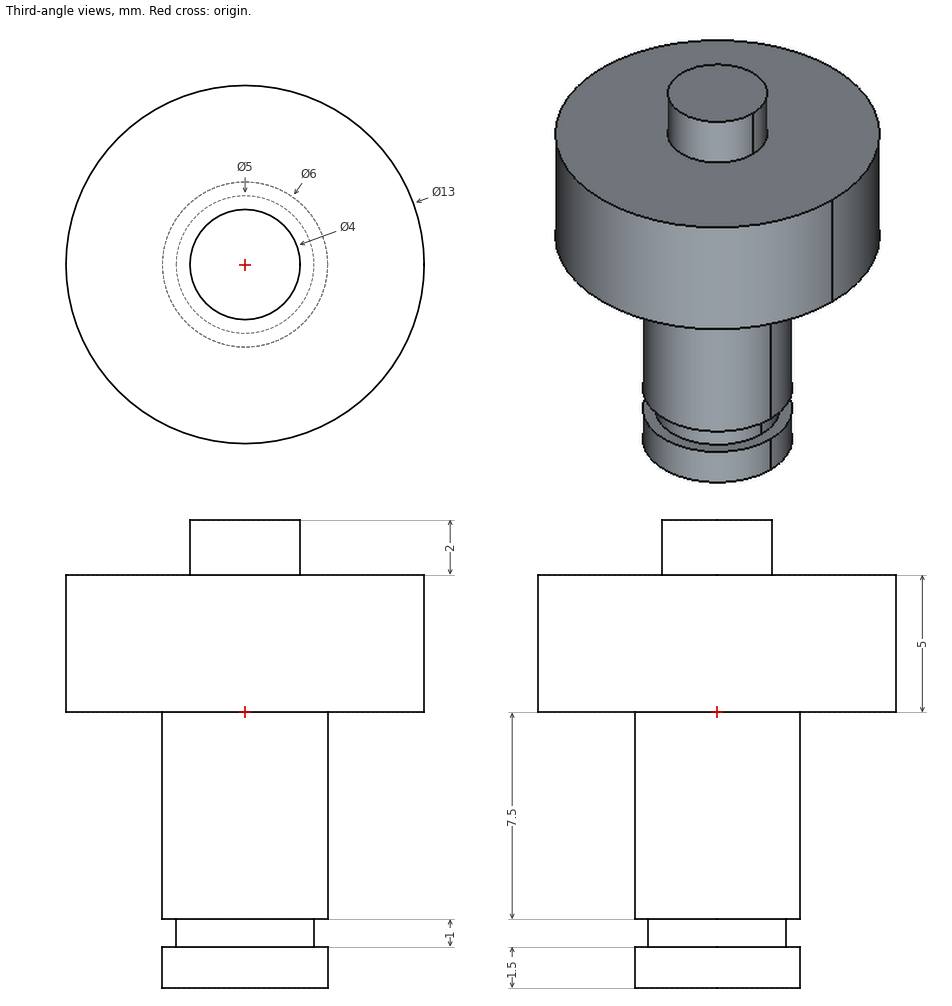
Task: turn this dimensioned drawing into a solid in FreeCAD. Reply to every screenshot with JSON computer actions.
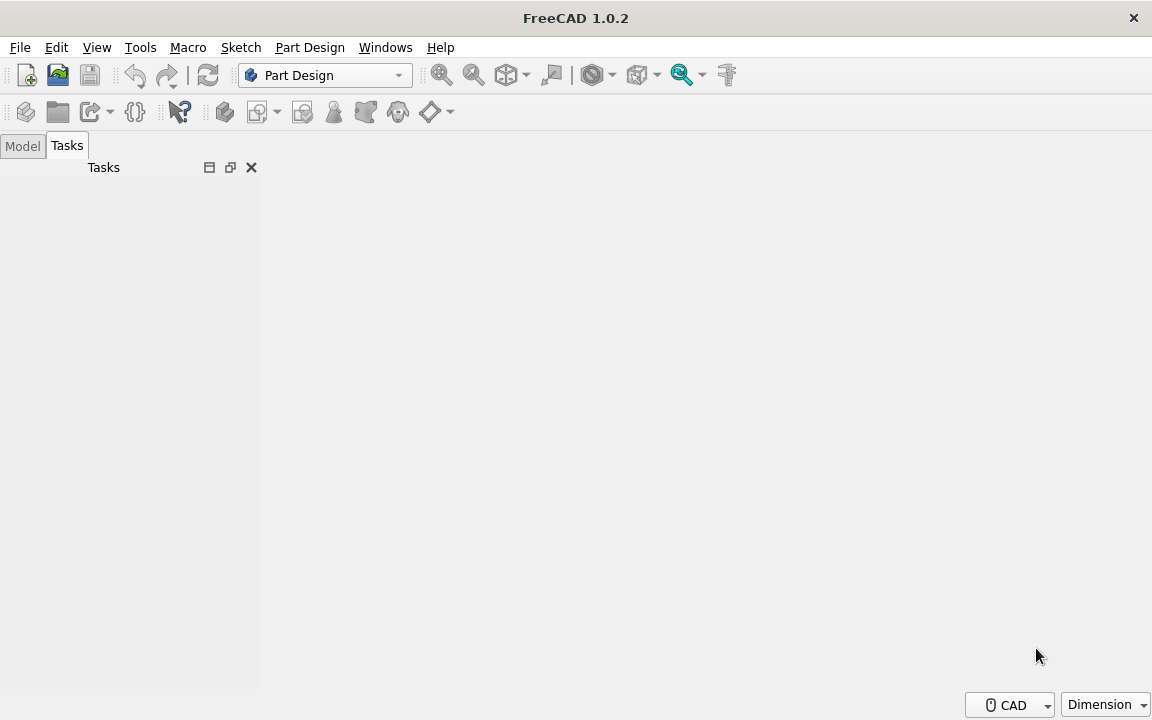
{"action": "key", "text": "ctrl+n"}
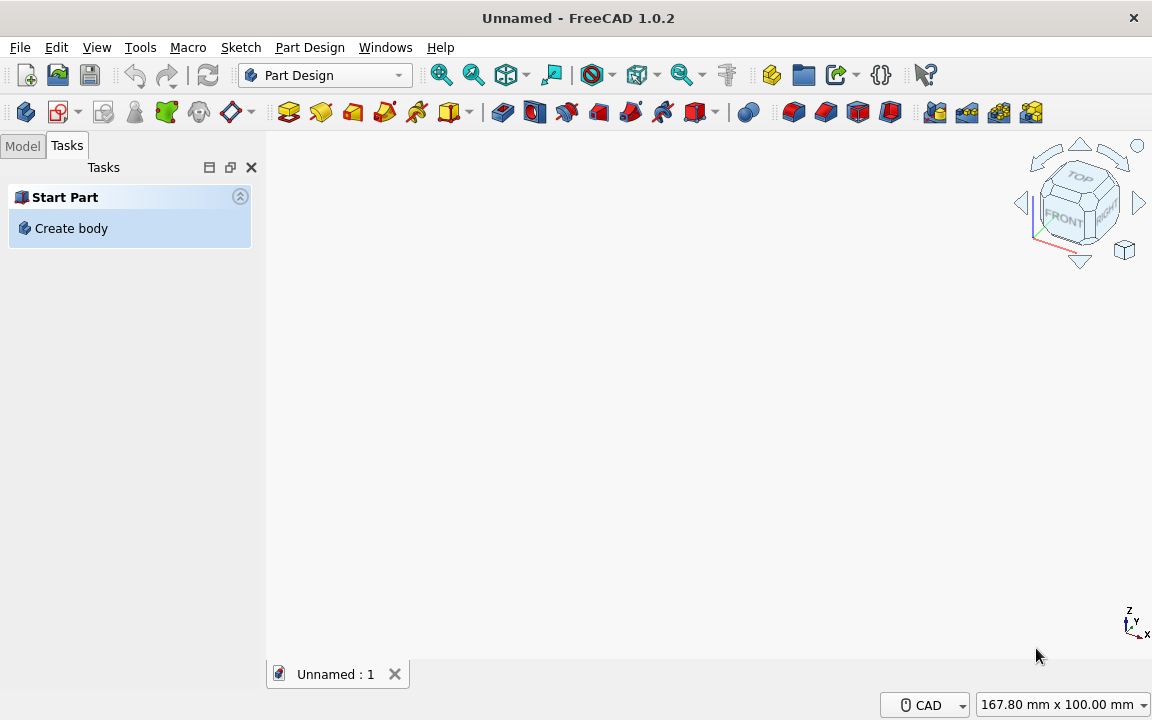
{"action": "left_click", "coordinate": [58, 112]}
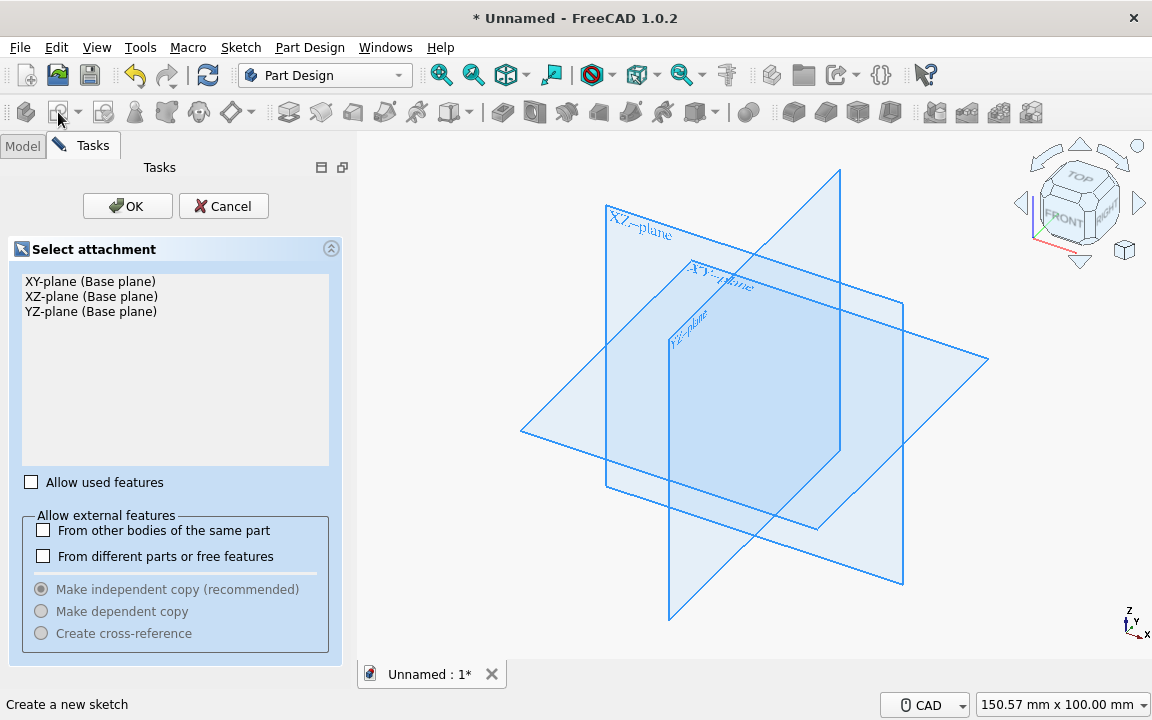
{"action": "left_click", "coordinate": [82, 282]}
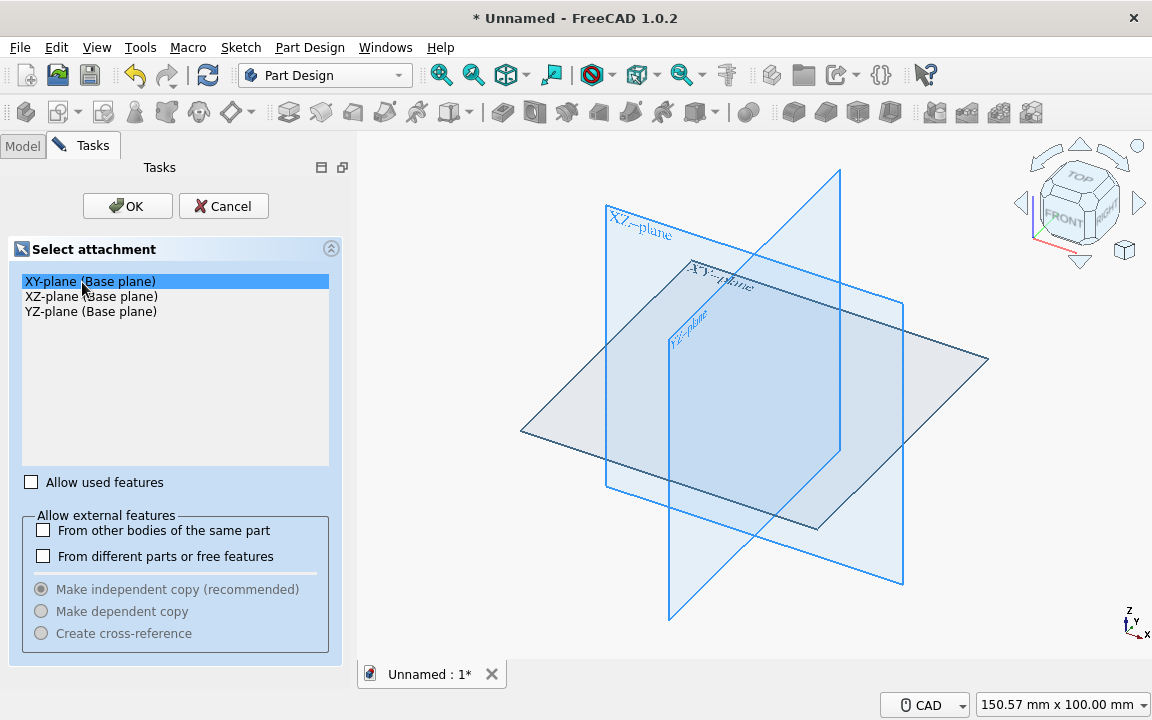
{"action": "left_click", "coordinate": [128, 206]}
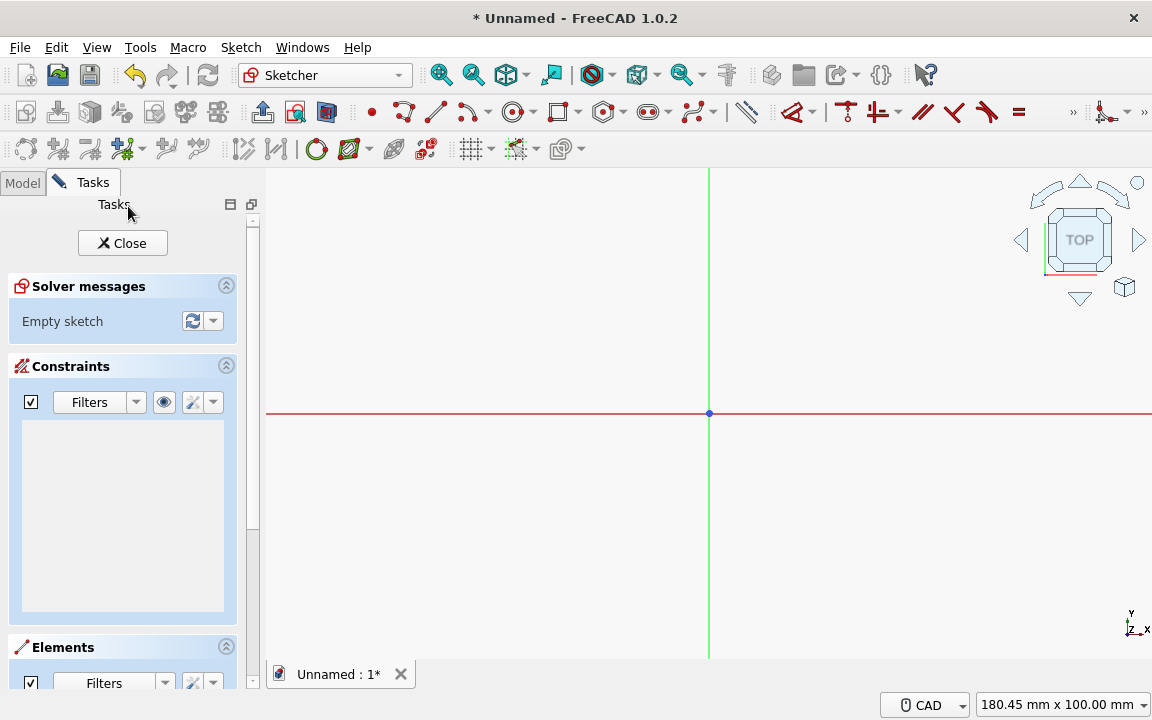
{"action": "scroll", "coordinate": [726, 414], "scroll_direction": "up", "scroll_amount": 8}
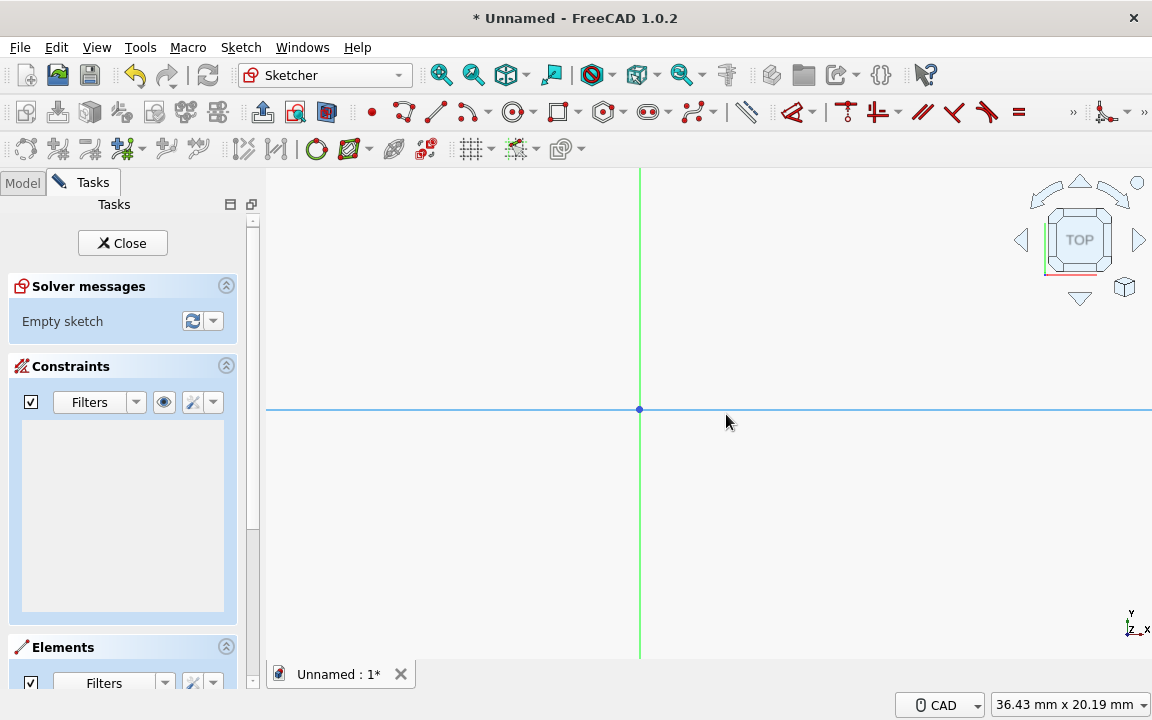
{"action": "key", "text": "g c"}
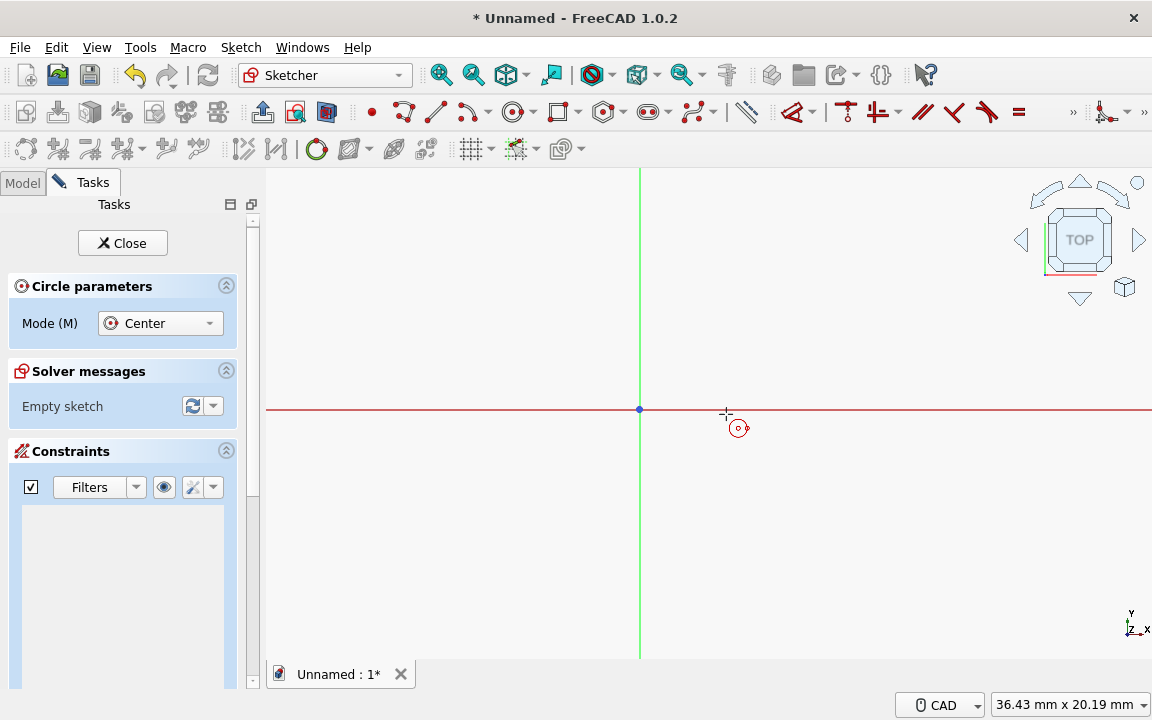
{"action": "left_click", "coordinate": [640, 410]}
{"action": "left_click", "coordinate": [752, 298]}
{"action": "key", "text": "Escape"}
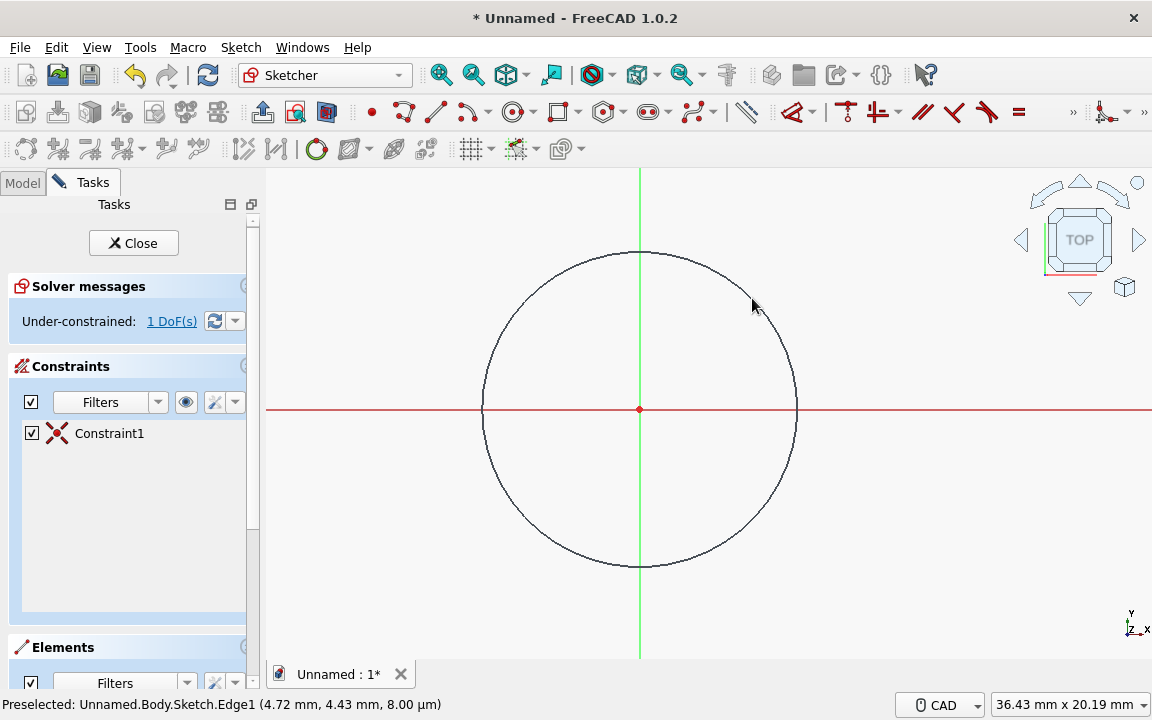
{"action": "key", "text": "d"}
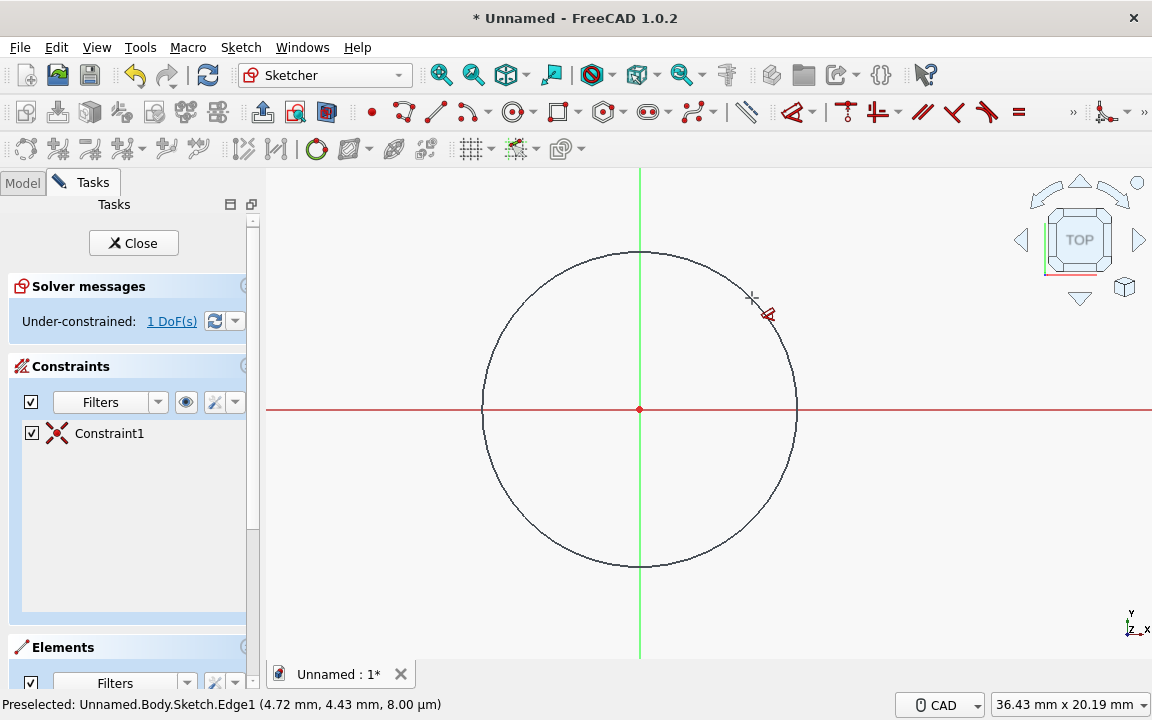
{"action": "left_click", "coordinate": [751, 298]}
{"action": "left_click", "coordinate": [774, 275]}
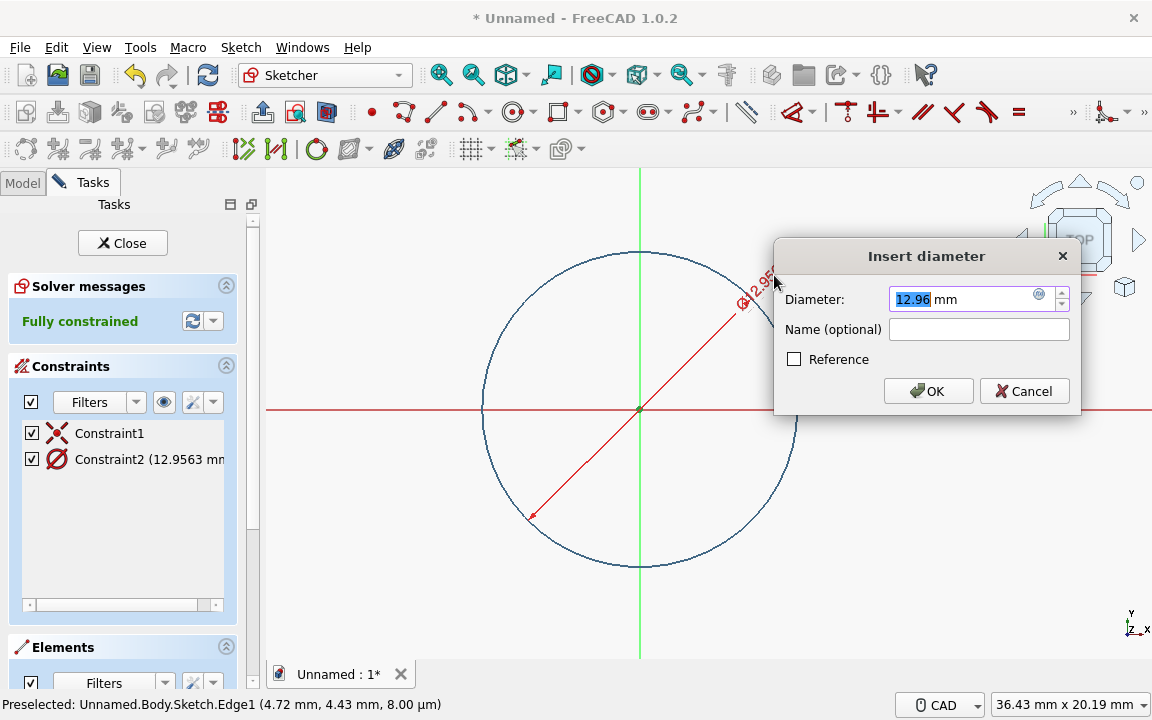
{"action": "type", "text": "13"}
{"action": "key", "text": "Return"}
{"action": "key", "text": "Escape"}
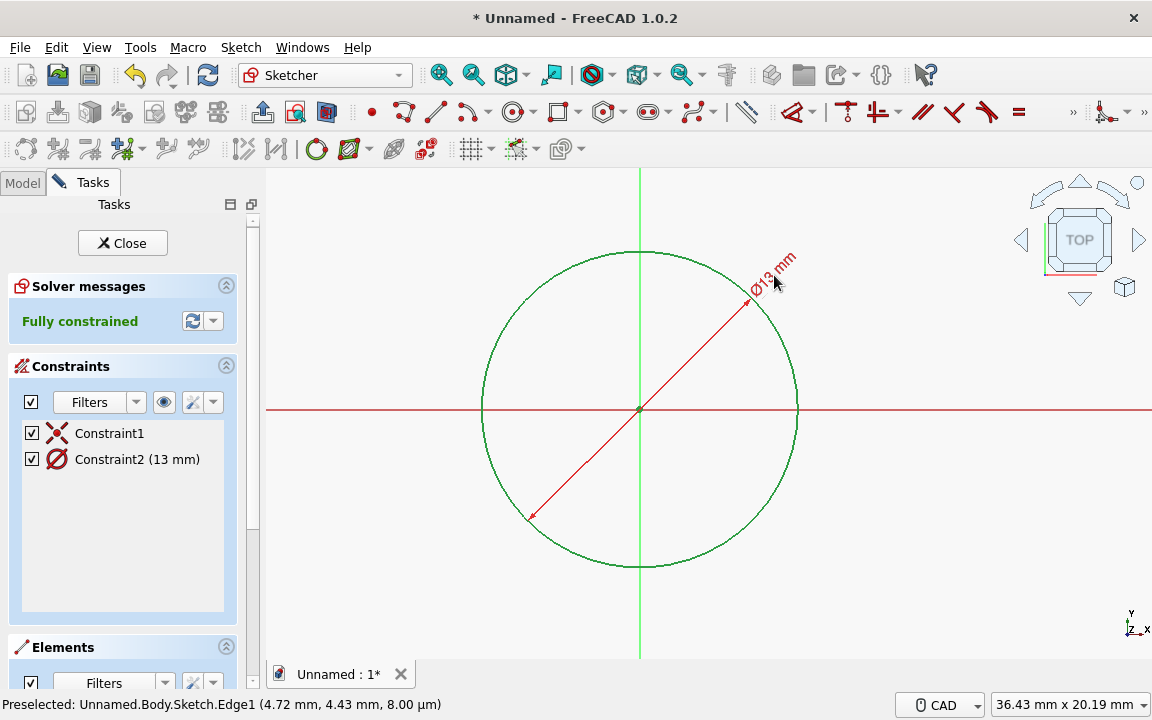
{"action": "left_click", "coordinate": [123, 243]}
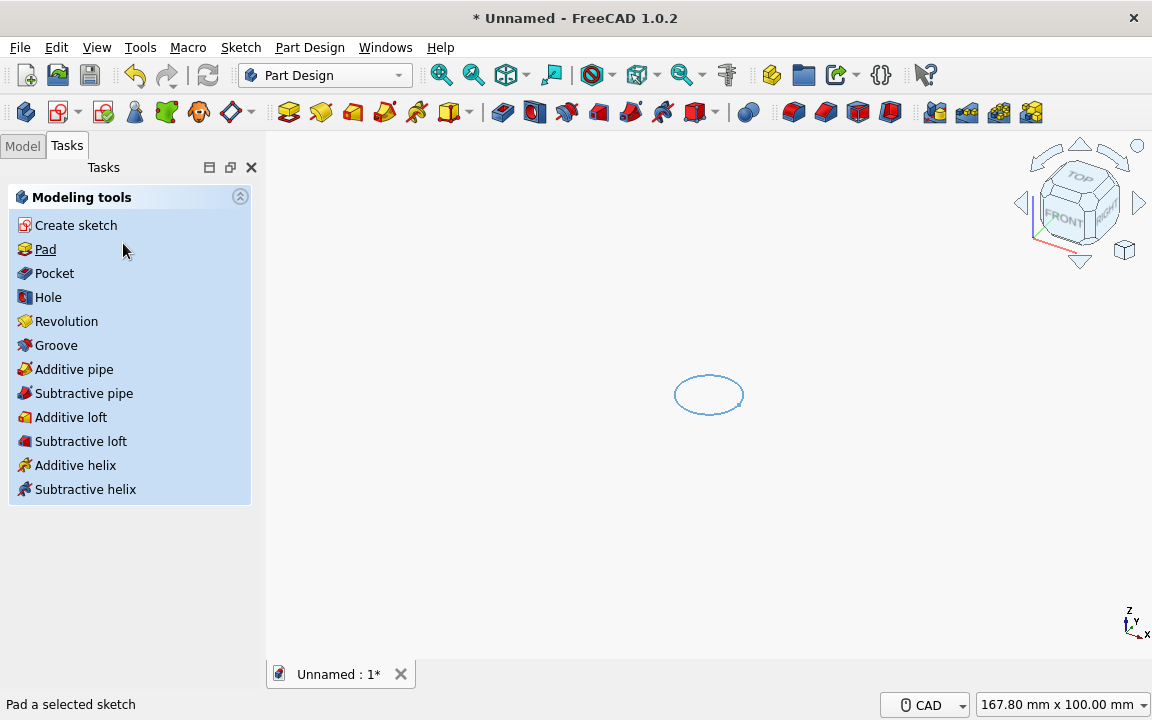
{"action": "left_click", "coordinate": [290, 112]}